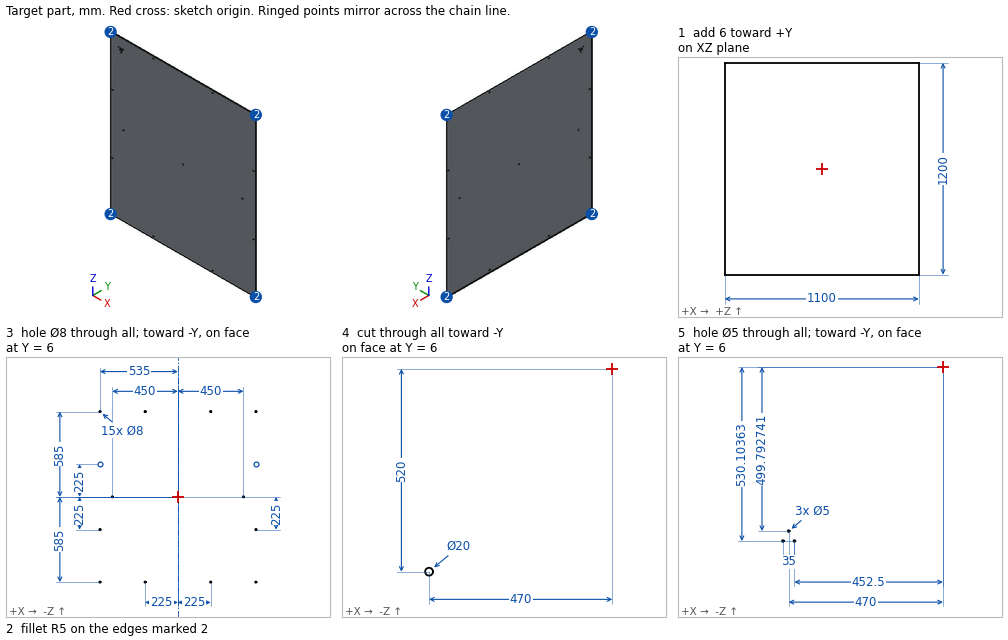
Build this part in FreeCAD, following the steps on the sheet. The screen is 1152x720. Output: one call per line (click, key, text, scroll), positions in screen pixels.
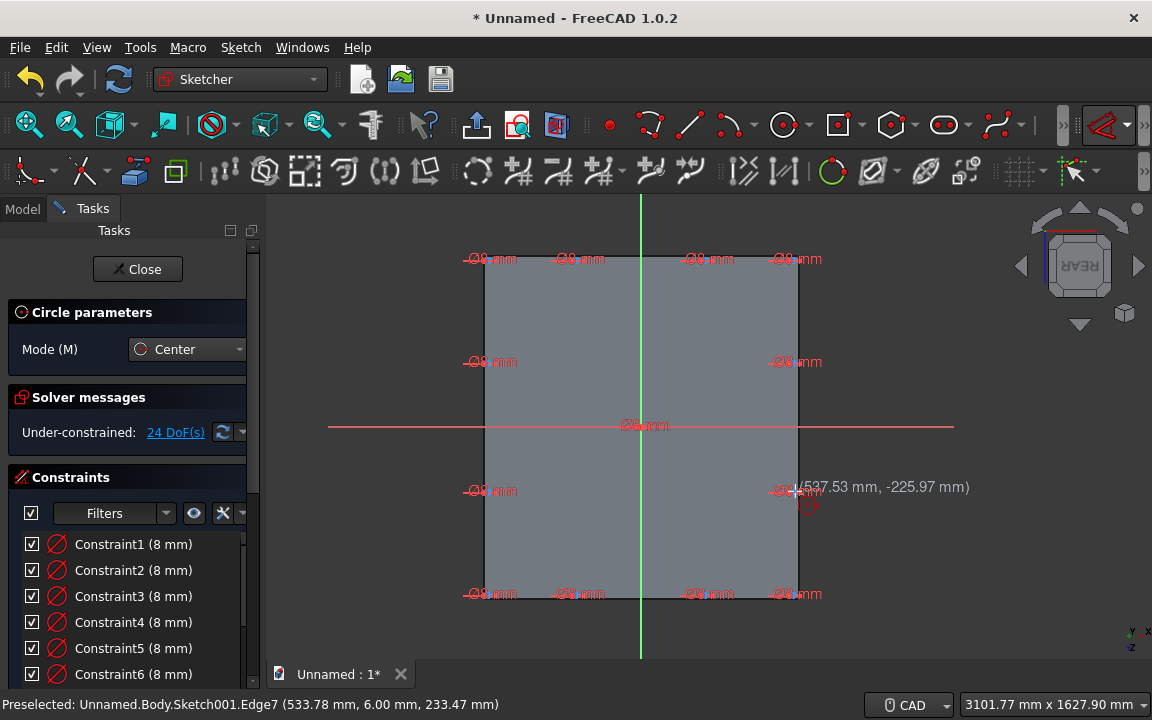
scroll(513, 427, up, 15)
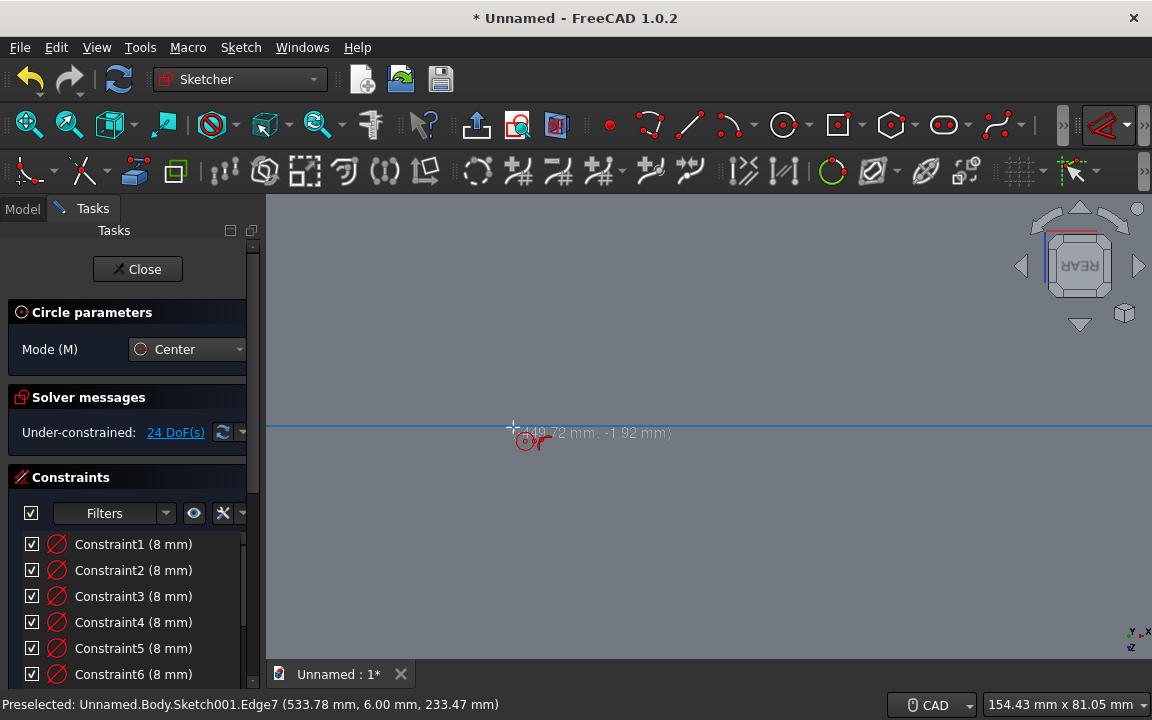
scroll(512, 427, down, 15)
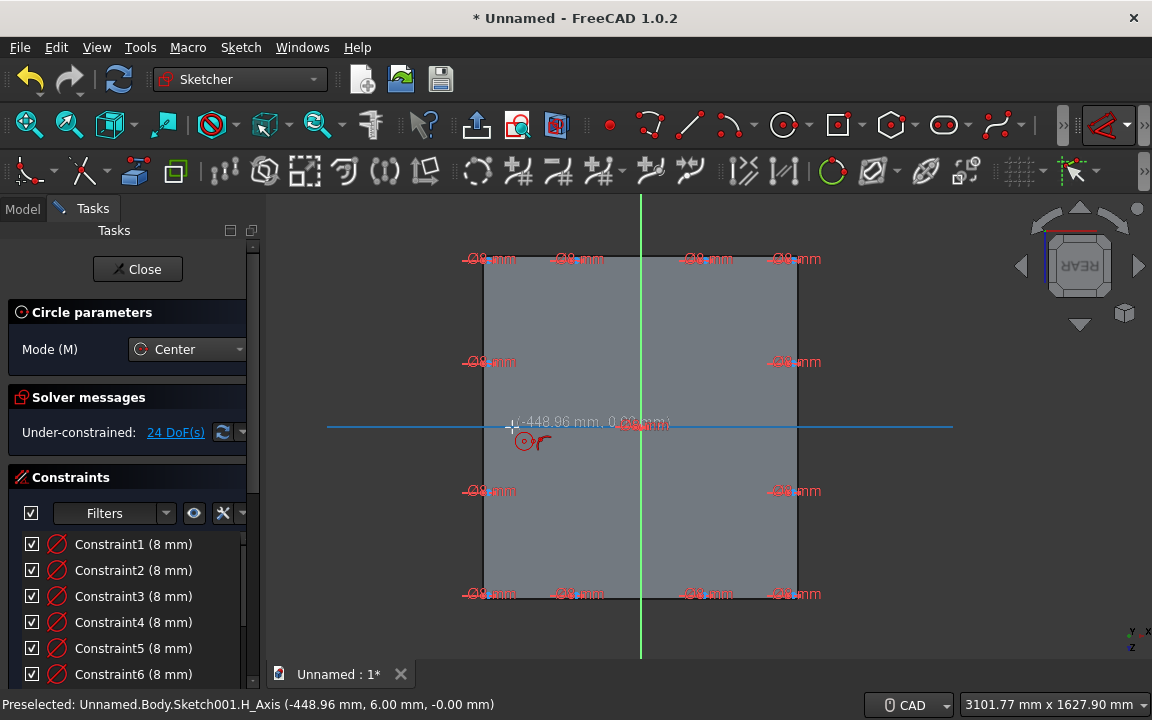
click(512, 427)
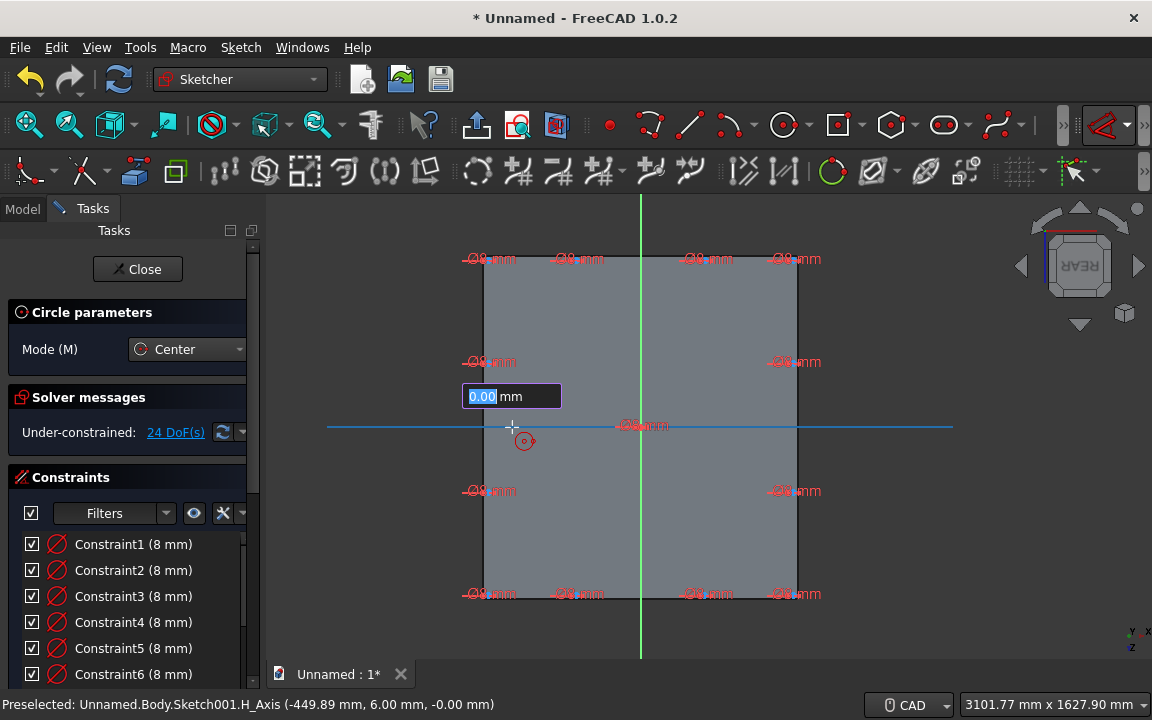
scroll(512, 426, up, 14)
move(514, 425)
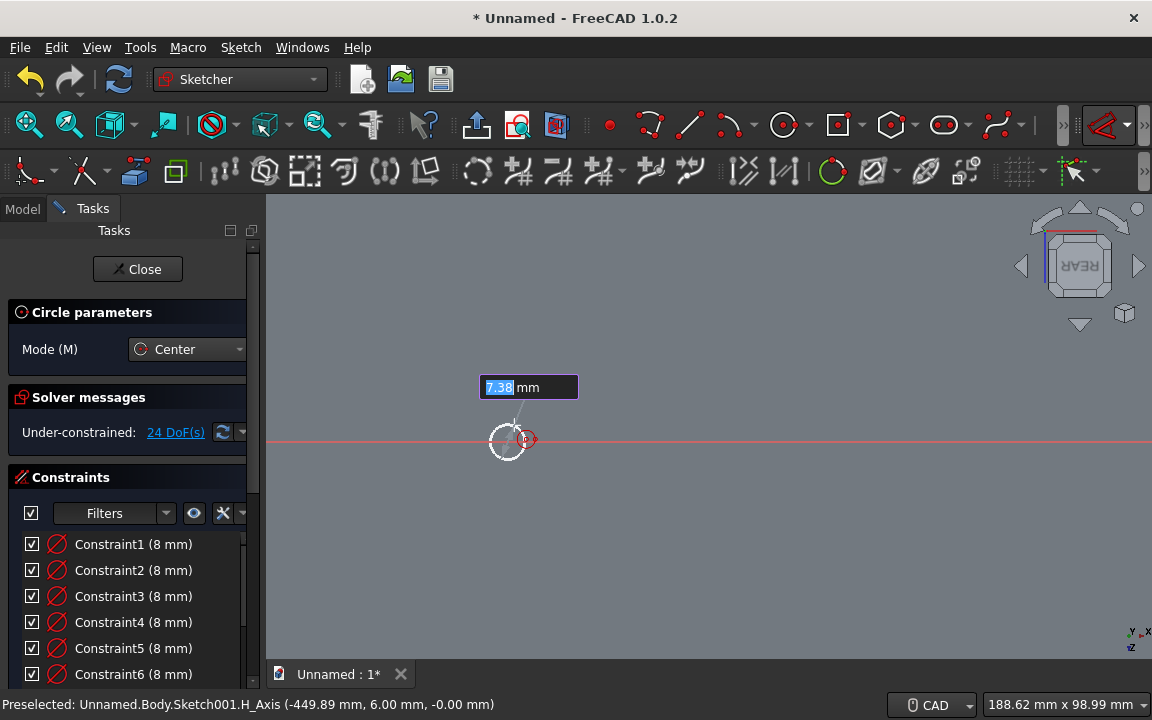
text(8)
key(Return)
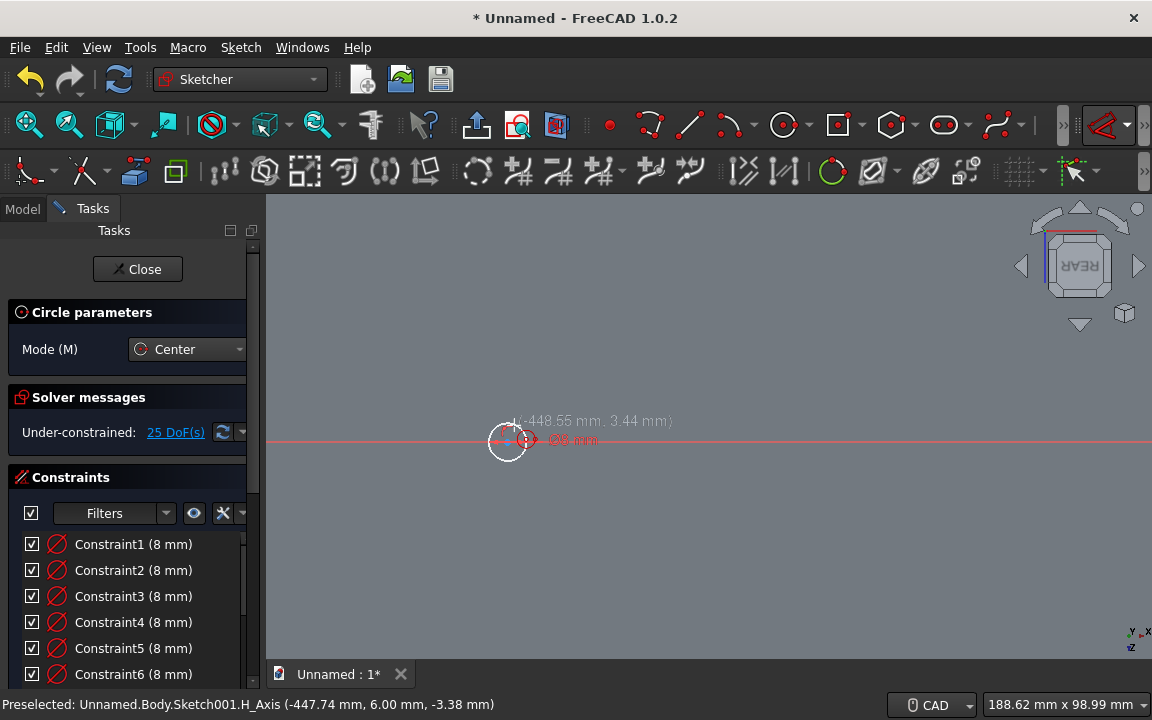
scroll(537, 426, down, 15)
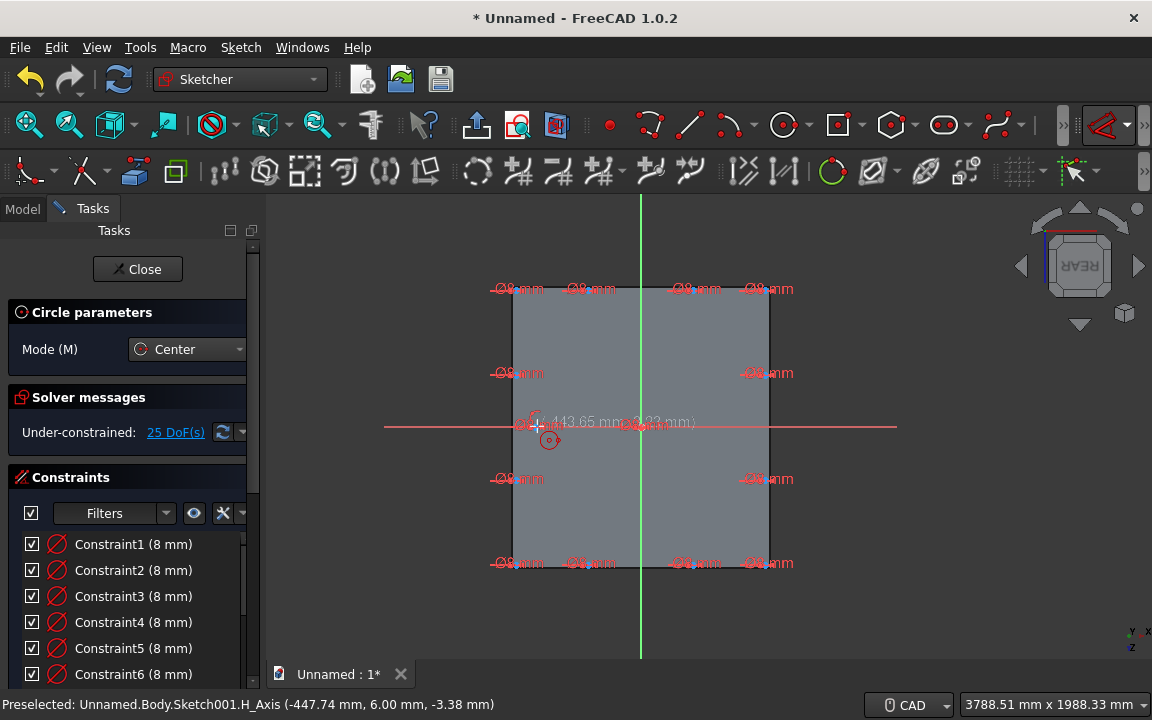
scroll(746, 427, up, 16)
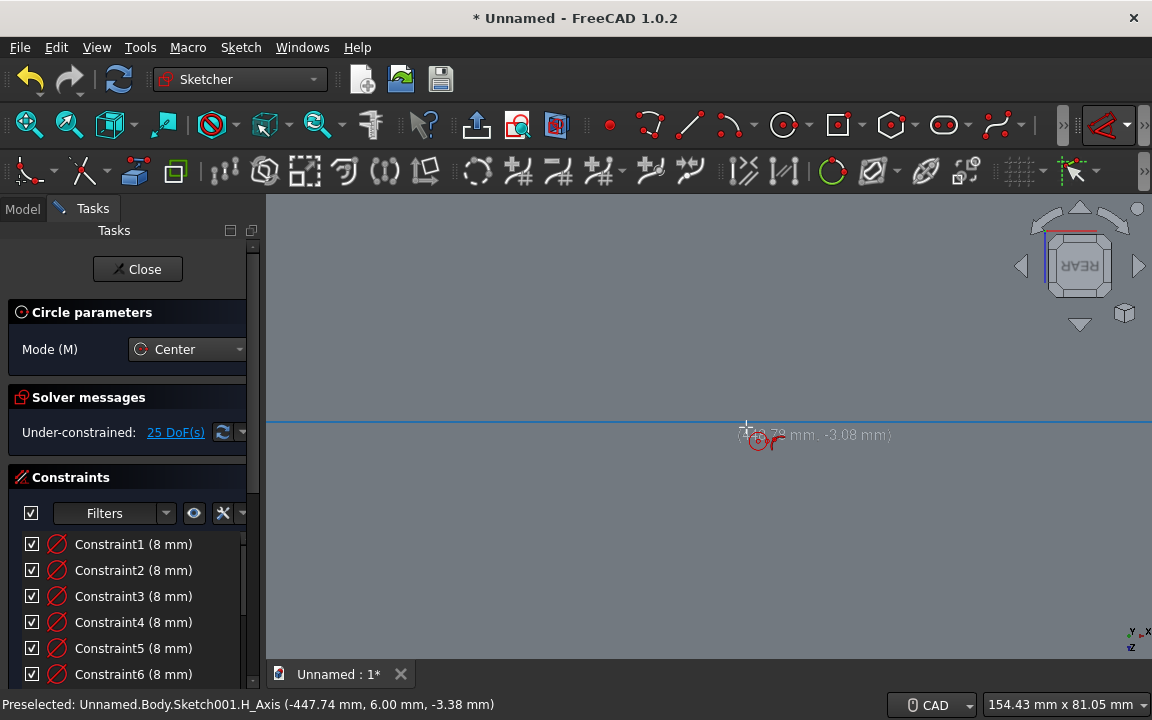
scroll(771, 427, down, 15)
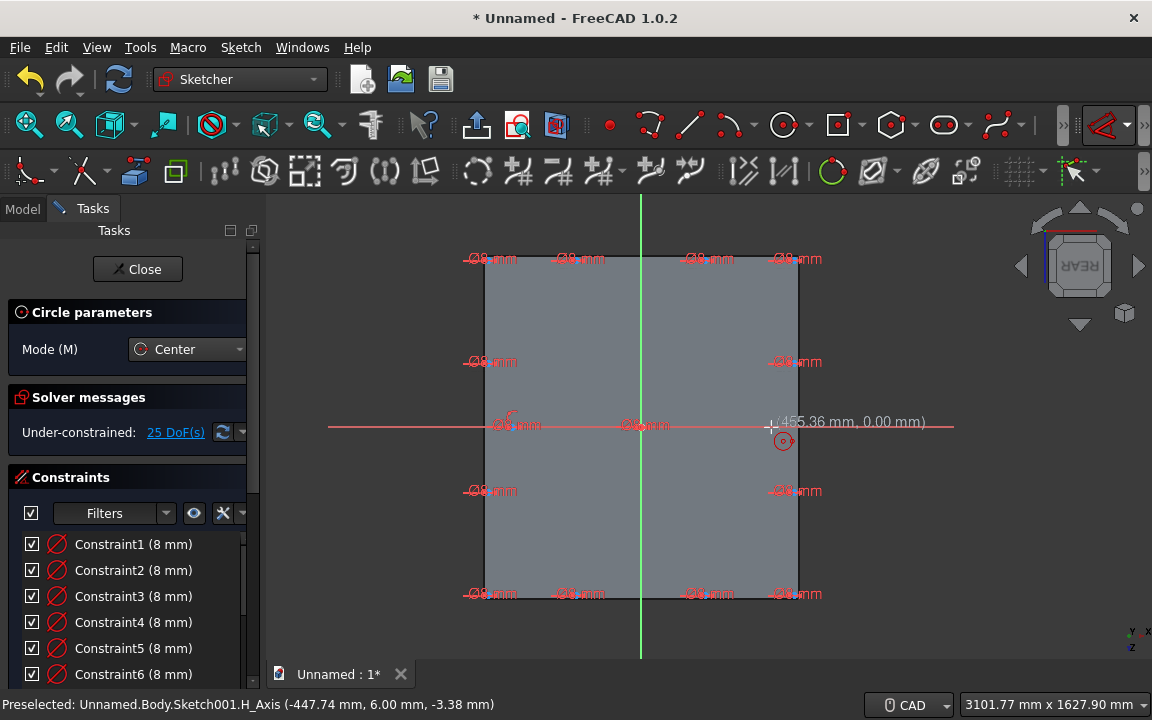
click(770, 427)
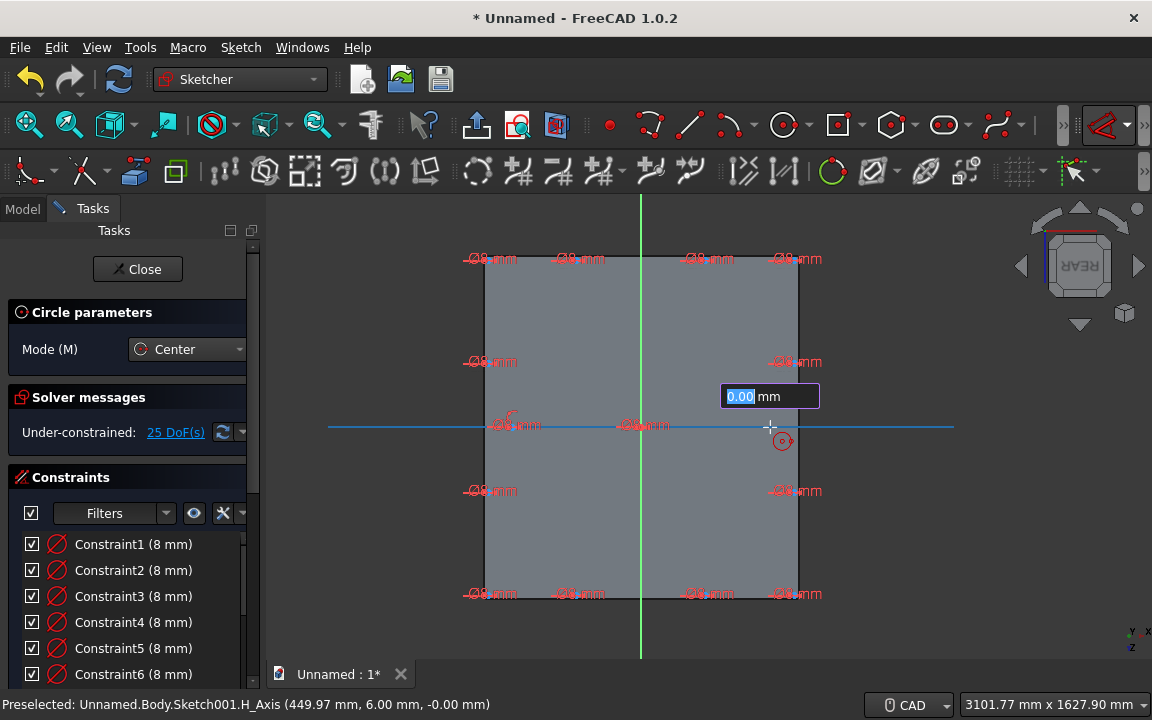
scroll(770, 426, up, 14)
move(768, 421)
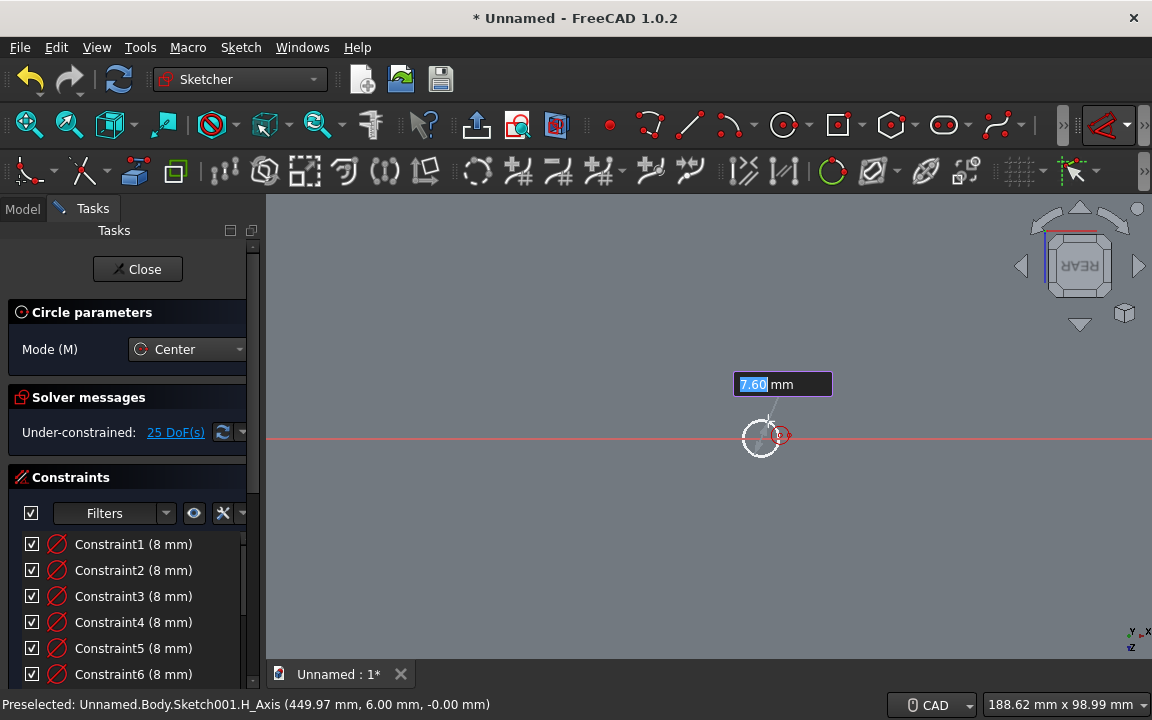
text(8)
key(Return)
key(Escape)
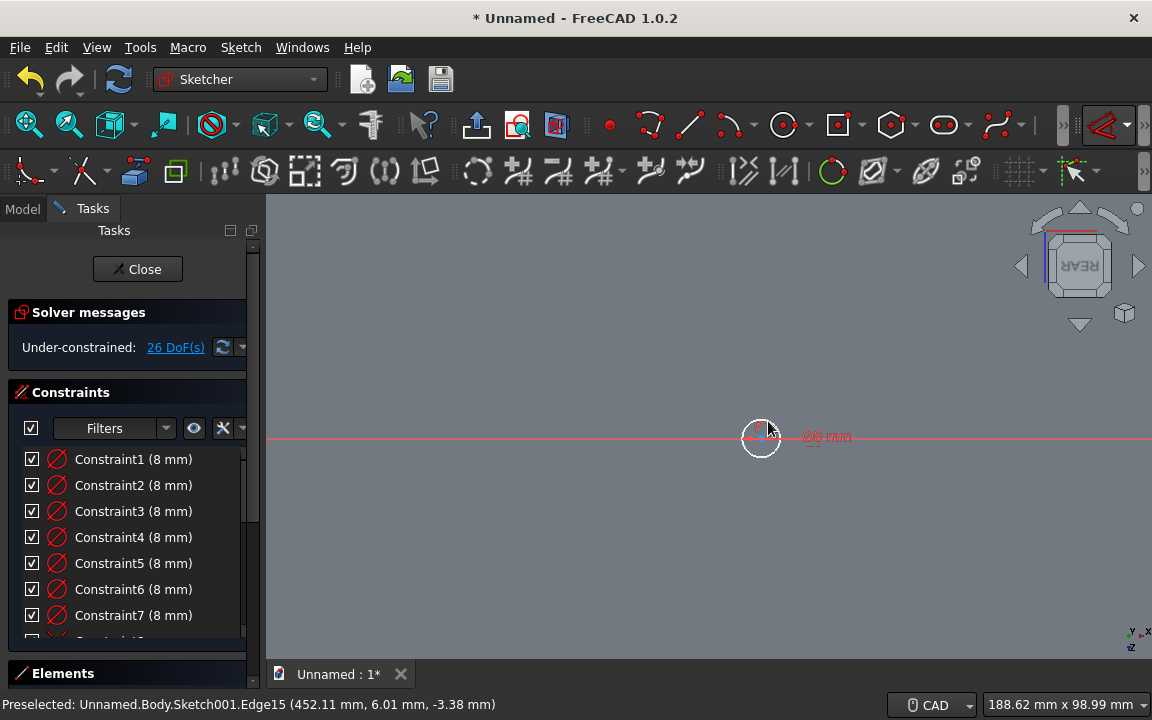
scroll(745, 426, down, 15)